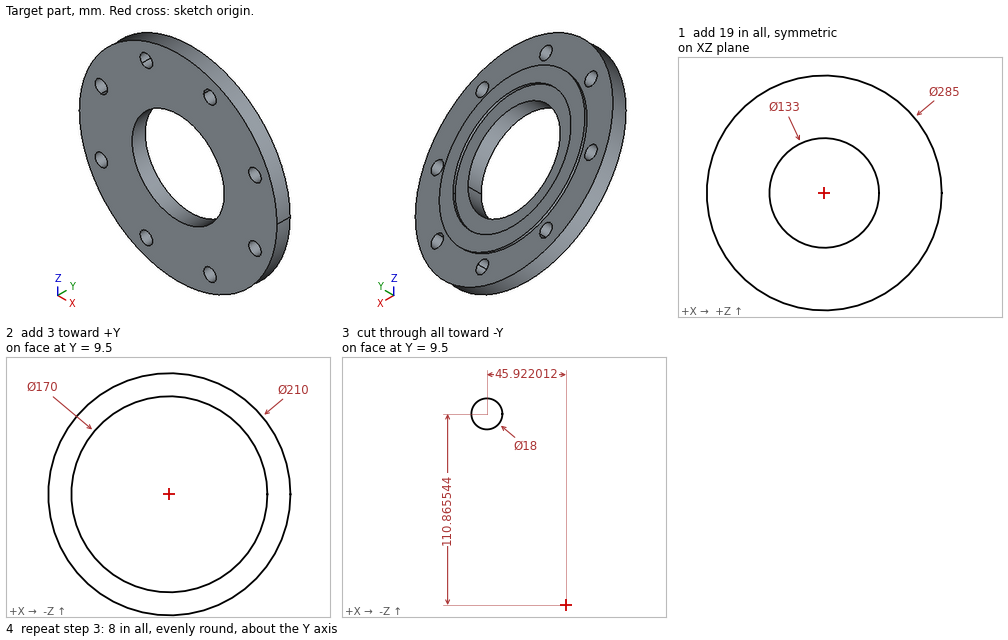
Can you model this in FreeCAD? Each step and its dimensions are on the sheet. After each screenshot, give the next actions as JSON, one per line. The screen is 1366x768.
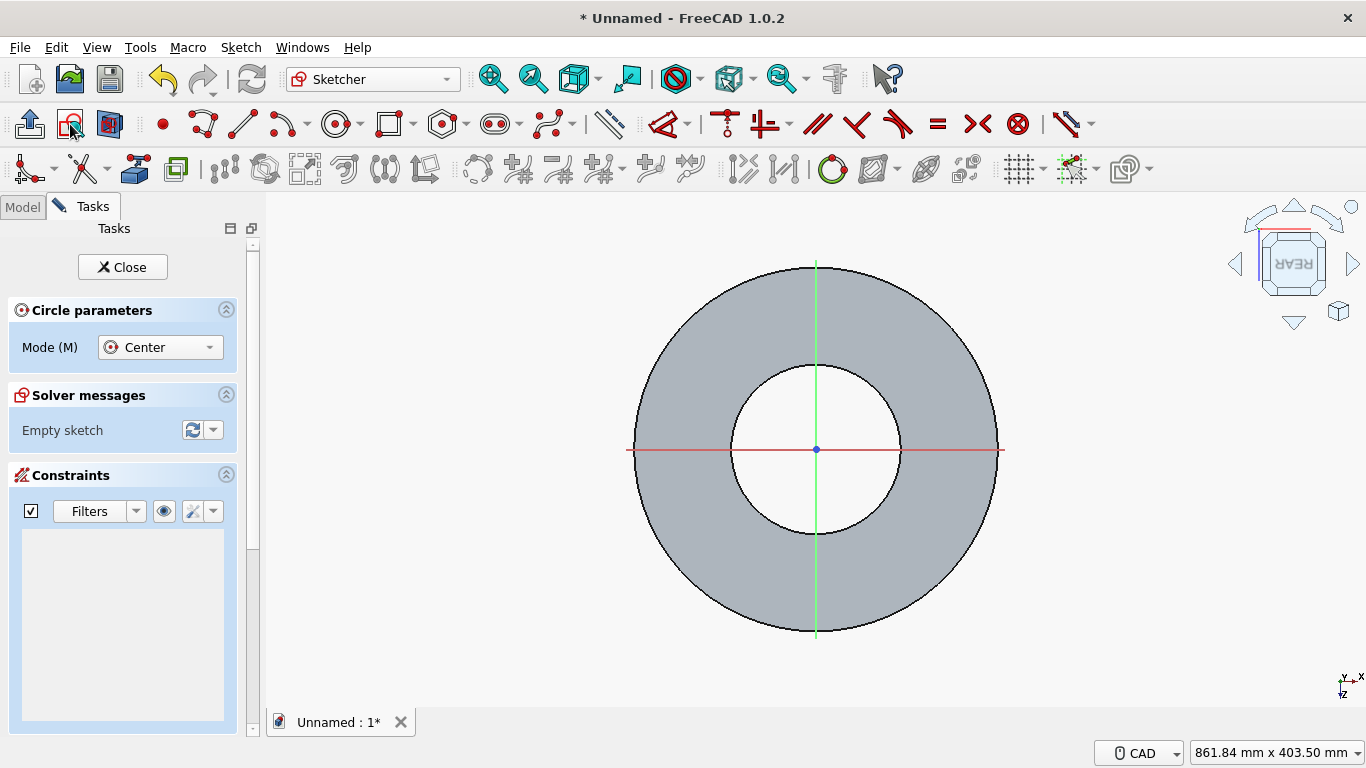
{"action": "left_click", "coordinate": [816, 449]}
{"action": "mouse_move", "coordinate": [911, 355]}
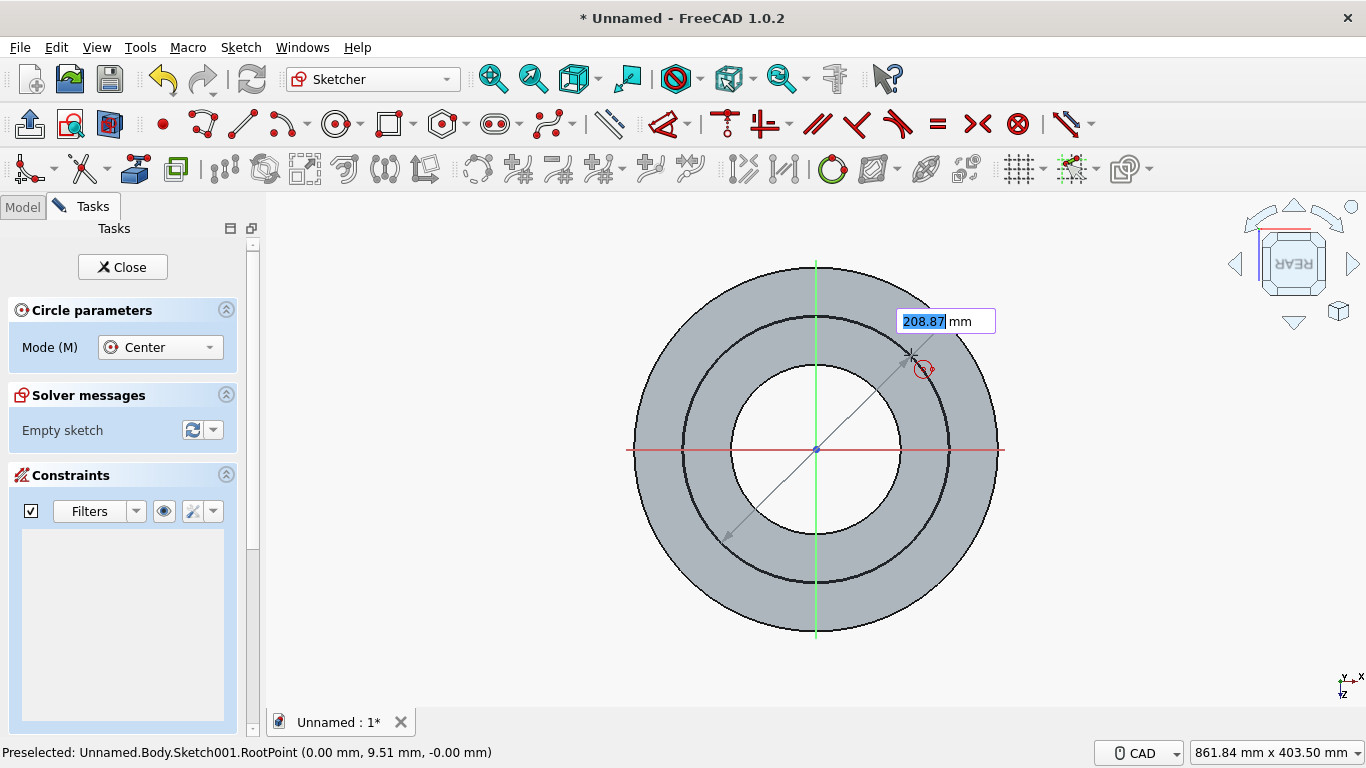
{"action": "type", "text": "210"}
{"action": "key", "text": "Return"}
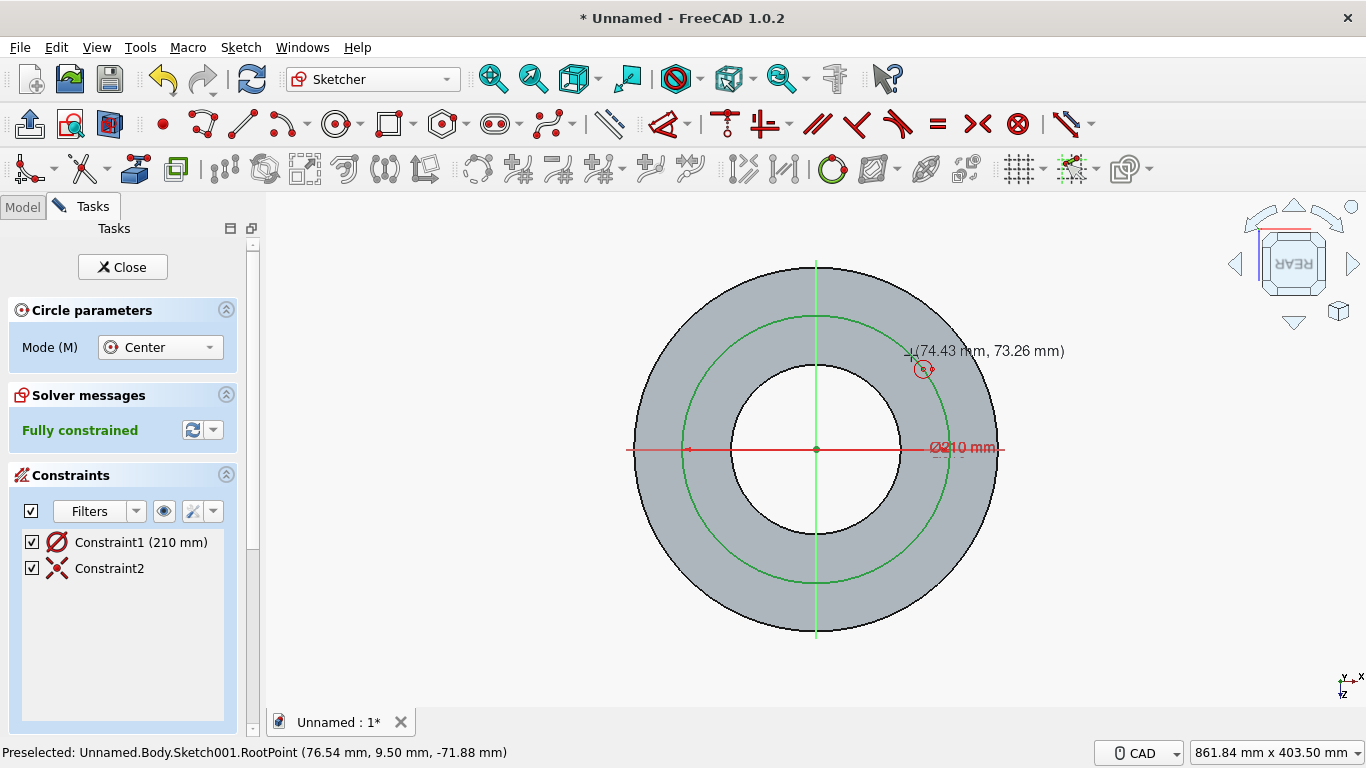
{"action": "left_click", "coordinate": [816, 449]}
{"action": "mouse_move", "coordinate": [893, 373]}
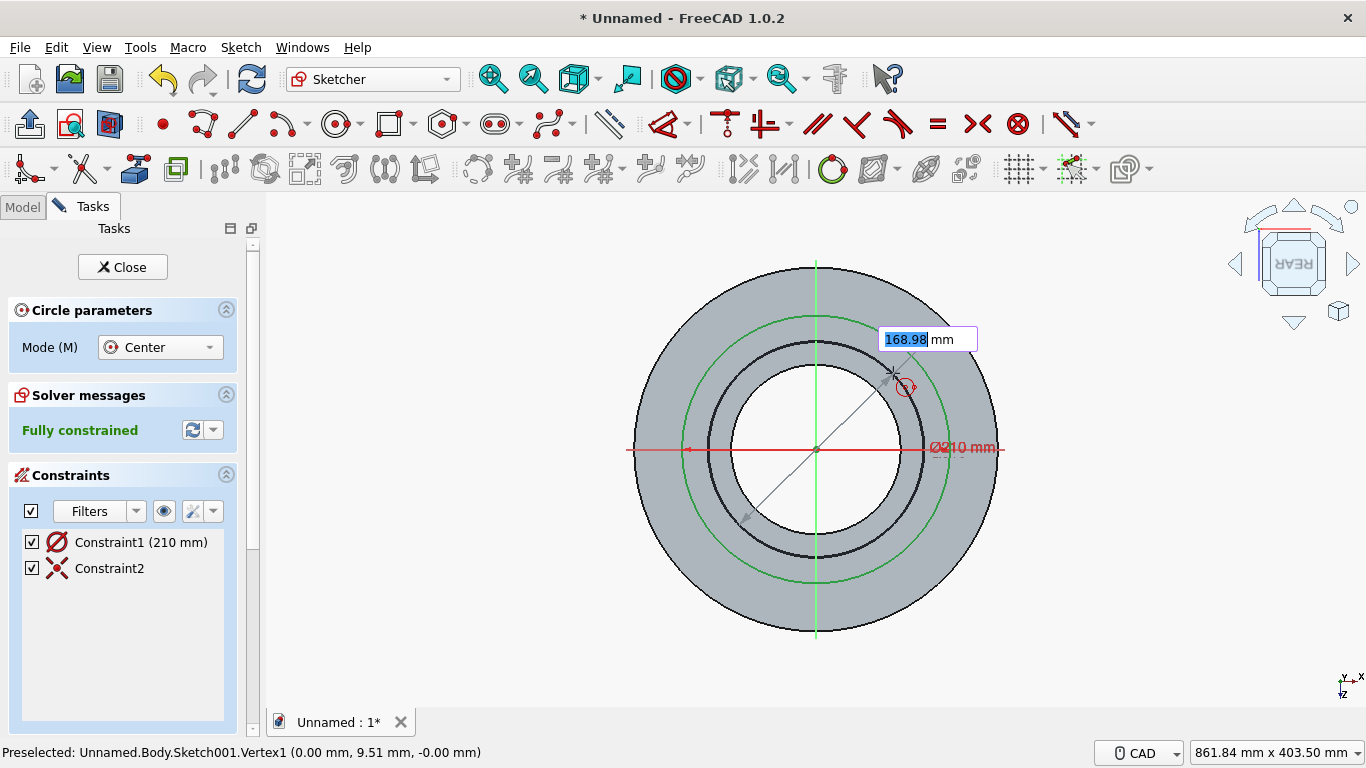
{"action": "type", "text": "170"}
{"action": "key", "text": "Return"}
{"action": "key", "text": "Escape"}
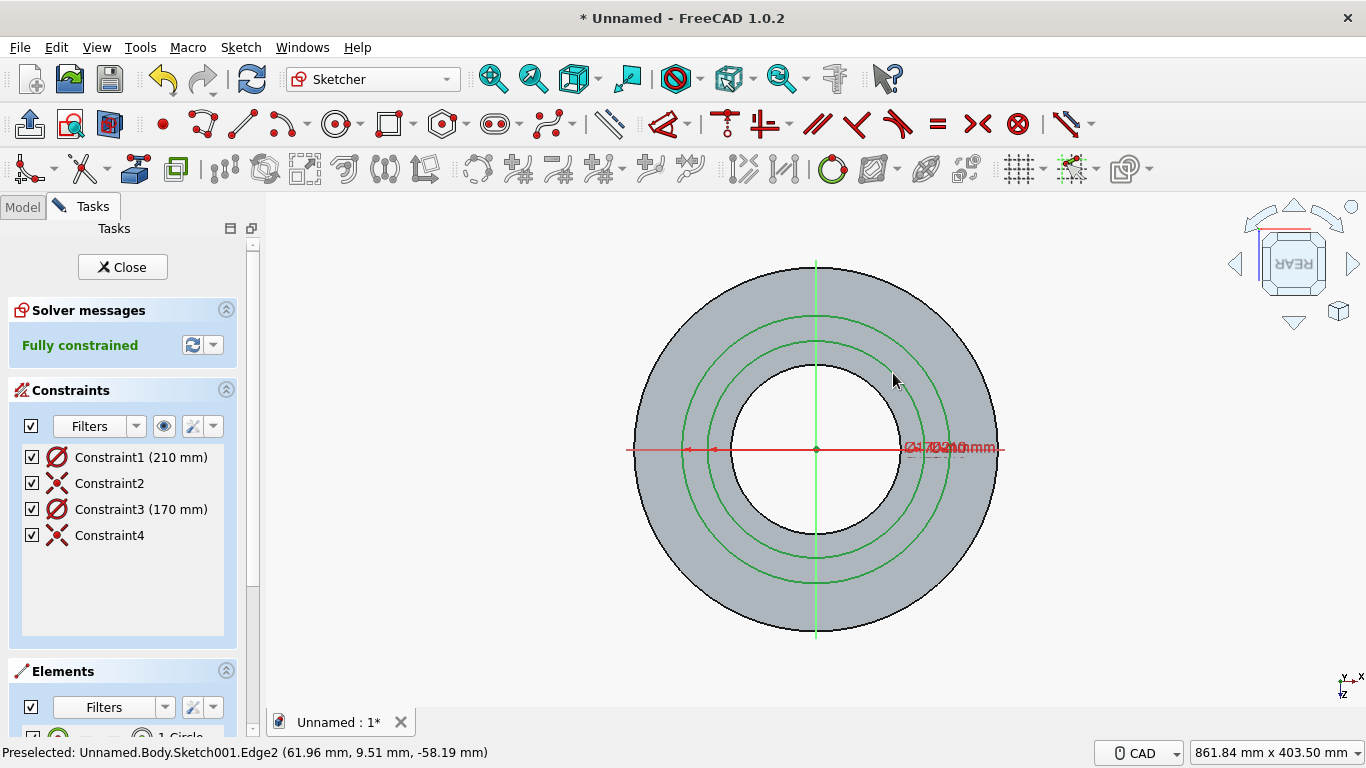
{"action": "left_click", "coordinate": [123, 267]}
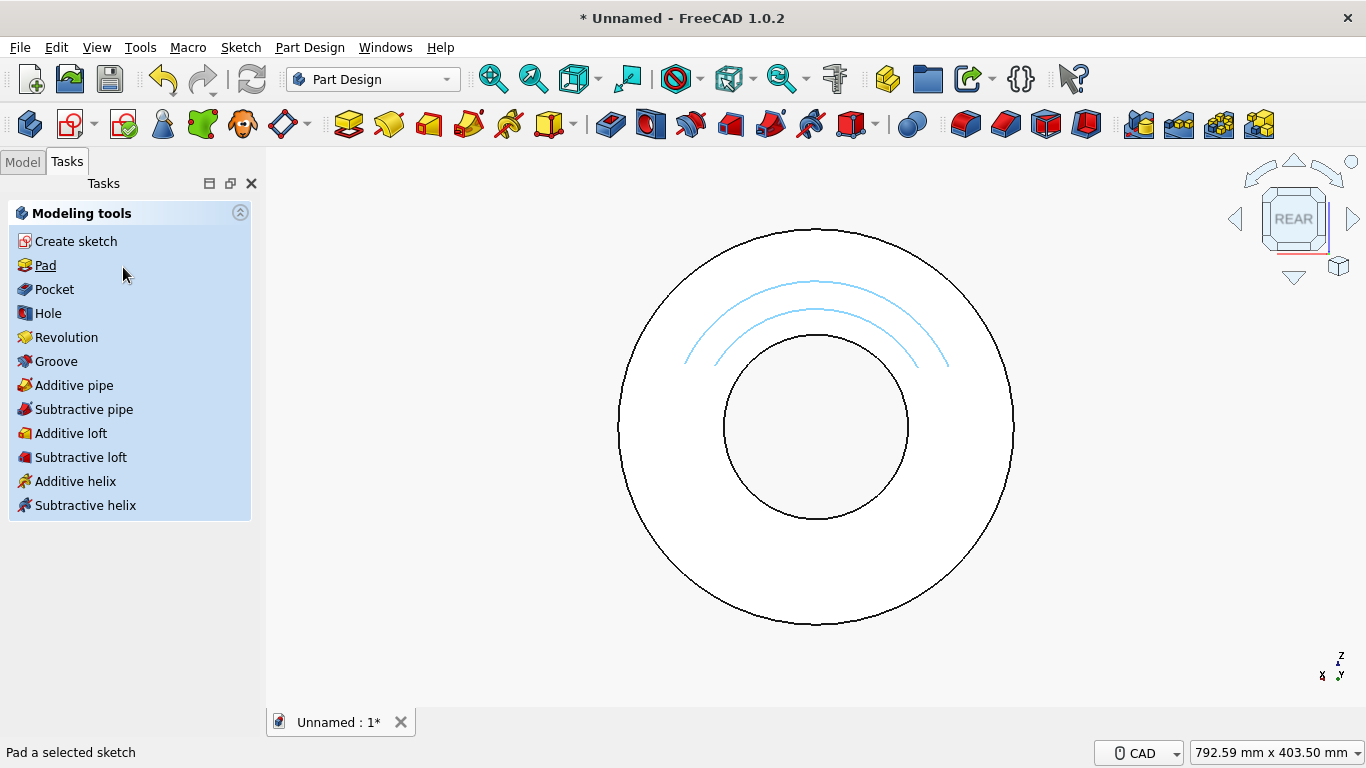
{"action": "left_click", "coordinate": [350, 124]}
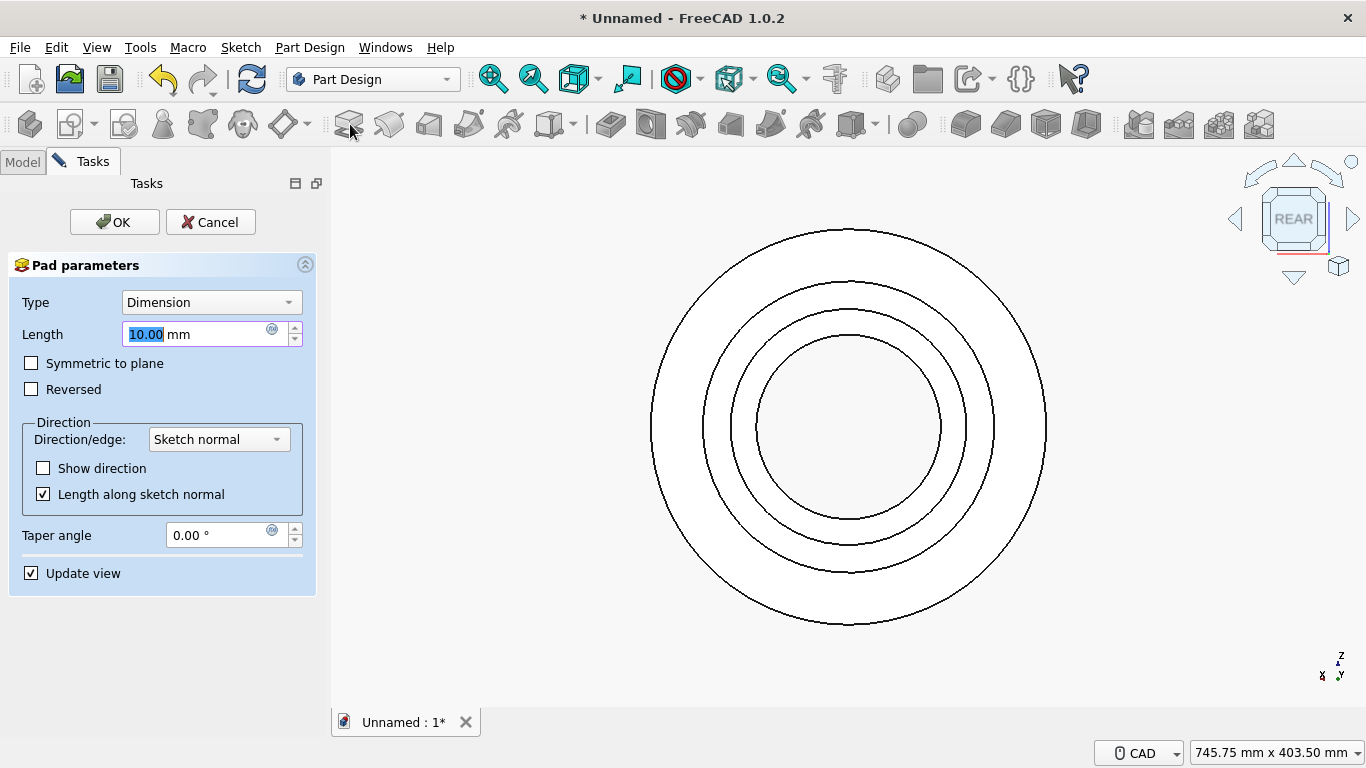
{"action": "type", "text": "3"}
{"action": "key", "text": "Tab"}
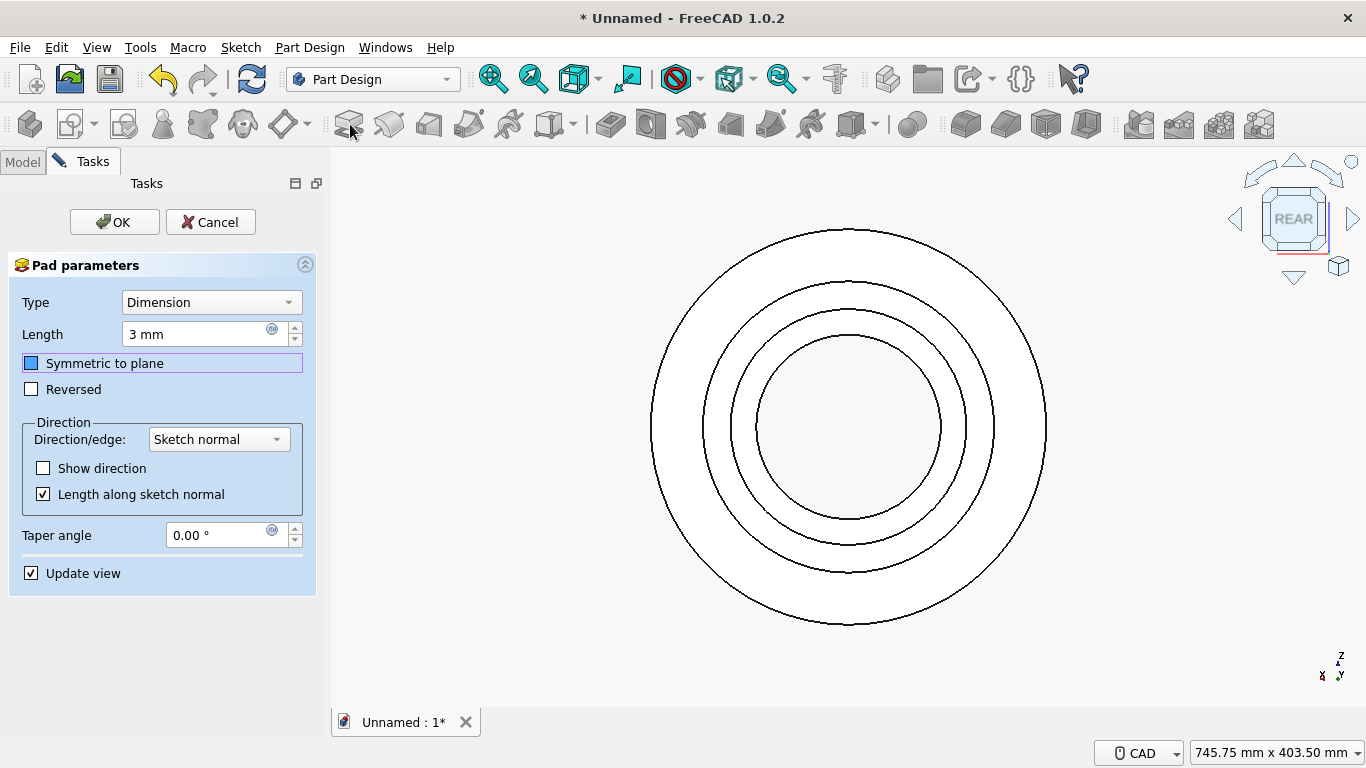
{"action": "left_click", "coordinate": [115, 222]}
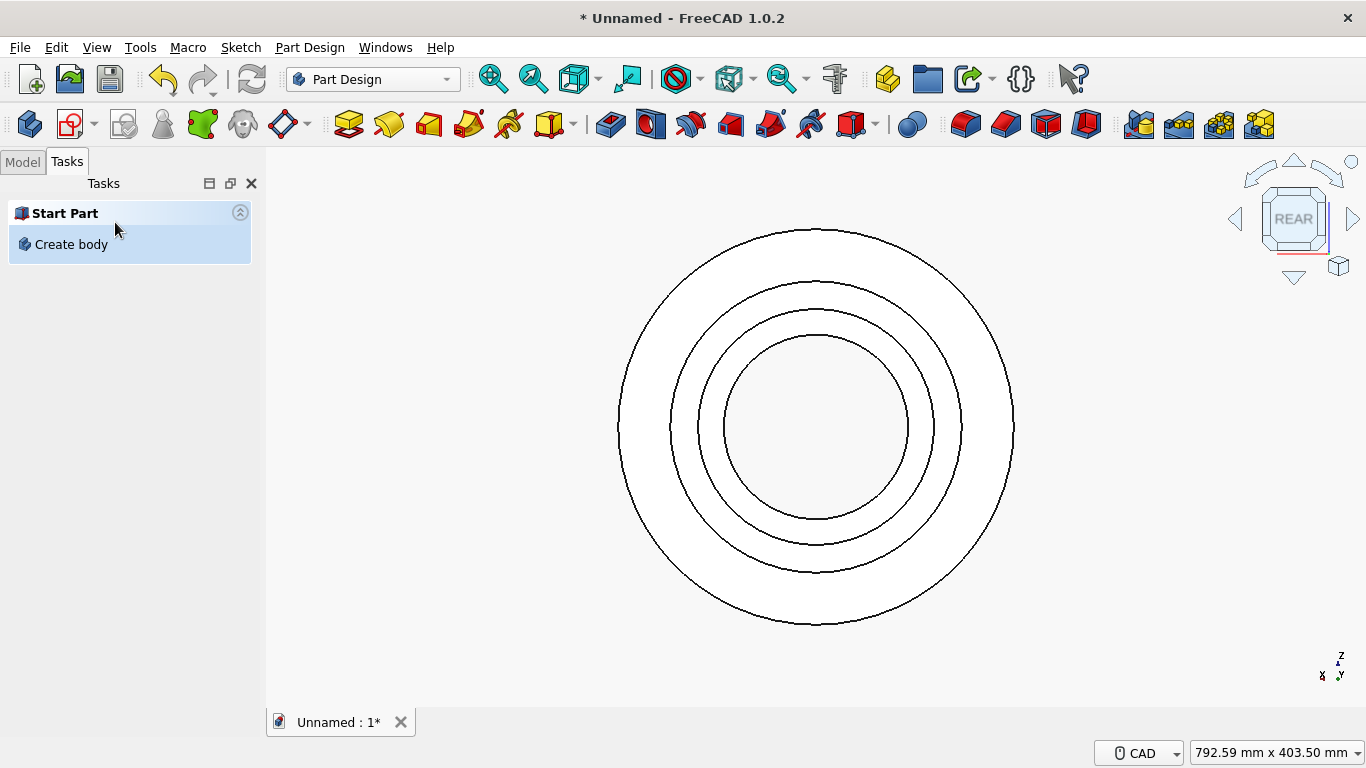
{"action": "left_click", "coordinate": [646, 426]}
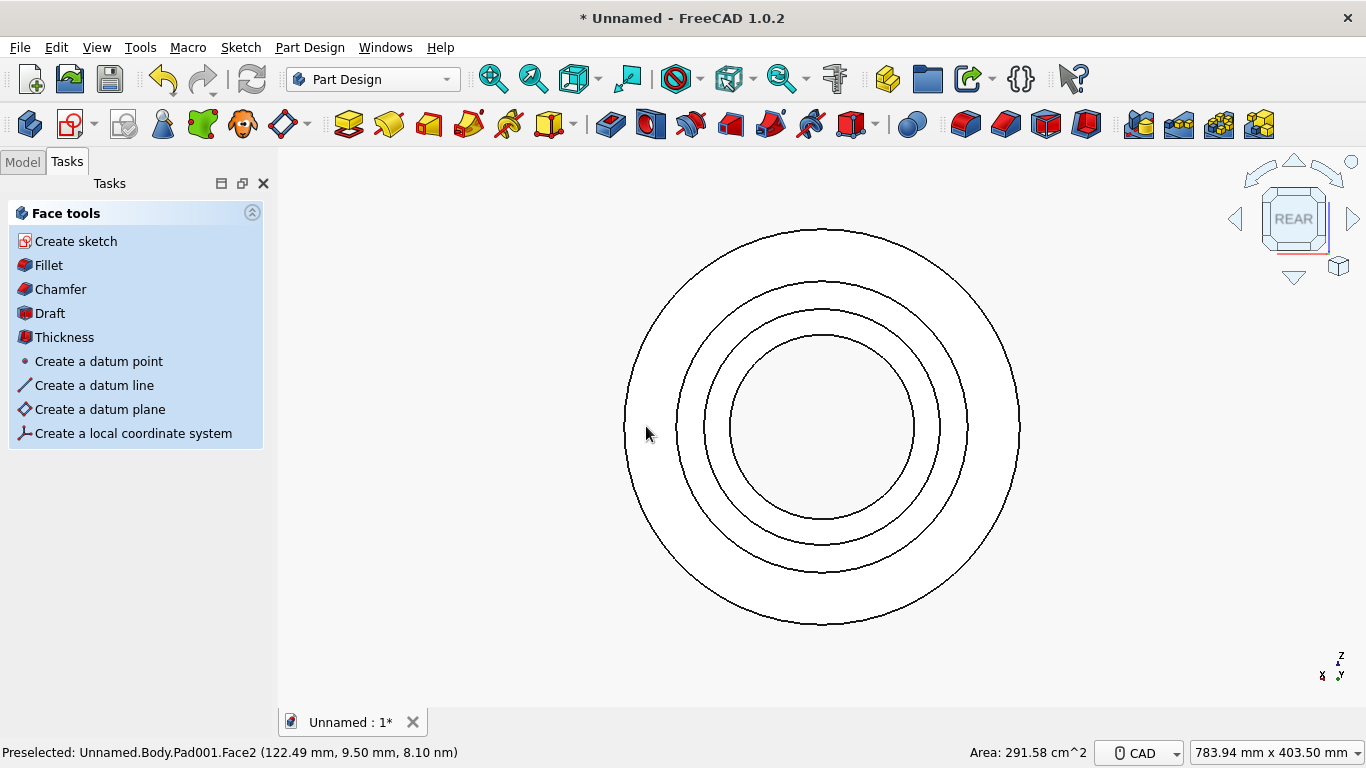
{"action": "left_click", "coordinate": [70, 124]}